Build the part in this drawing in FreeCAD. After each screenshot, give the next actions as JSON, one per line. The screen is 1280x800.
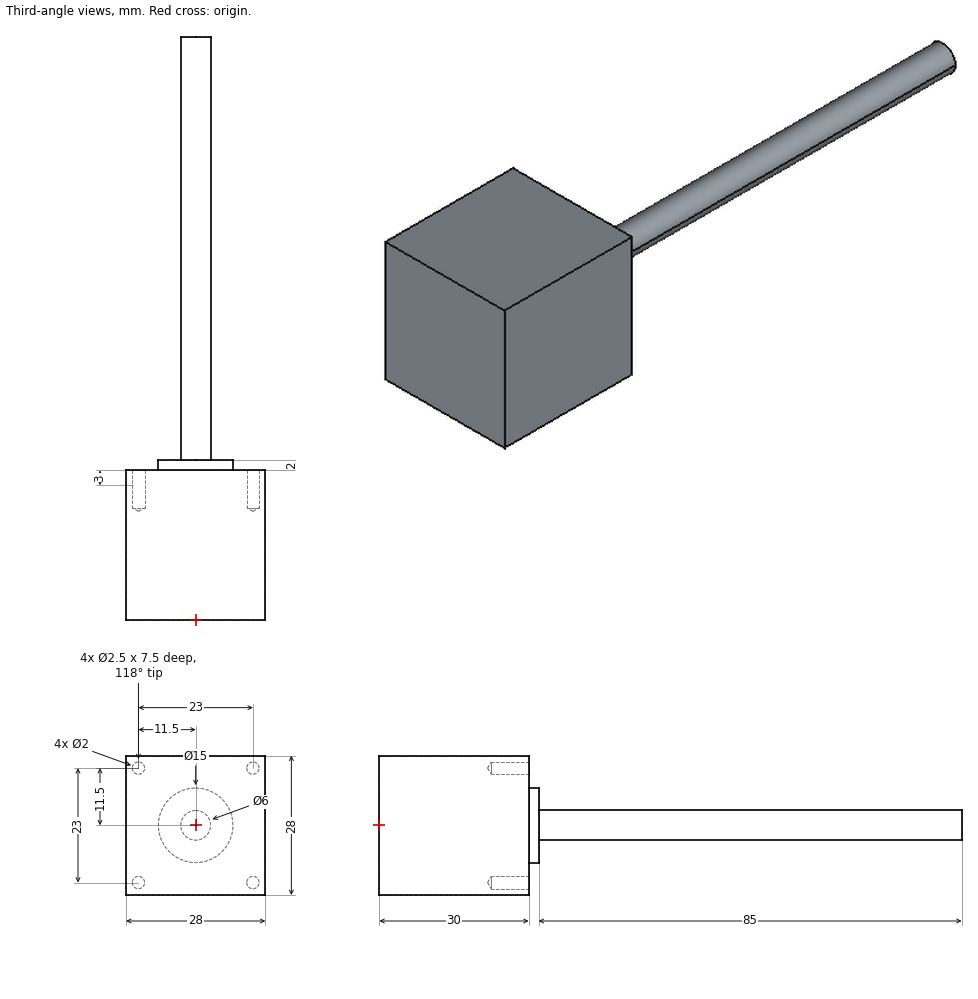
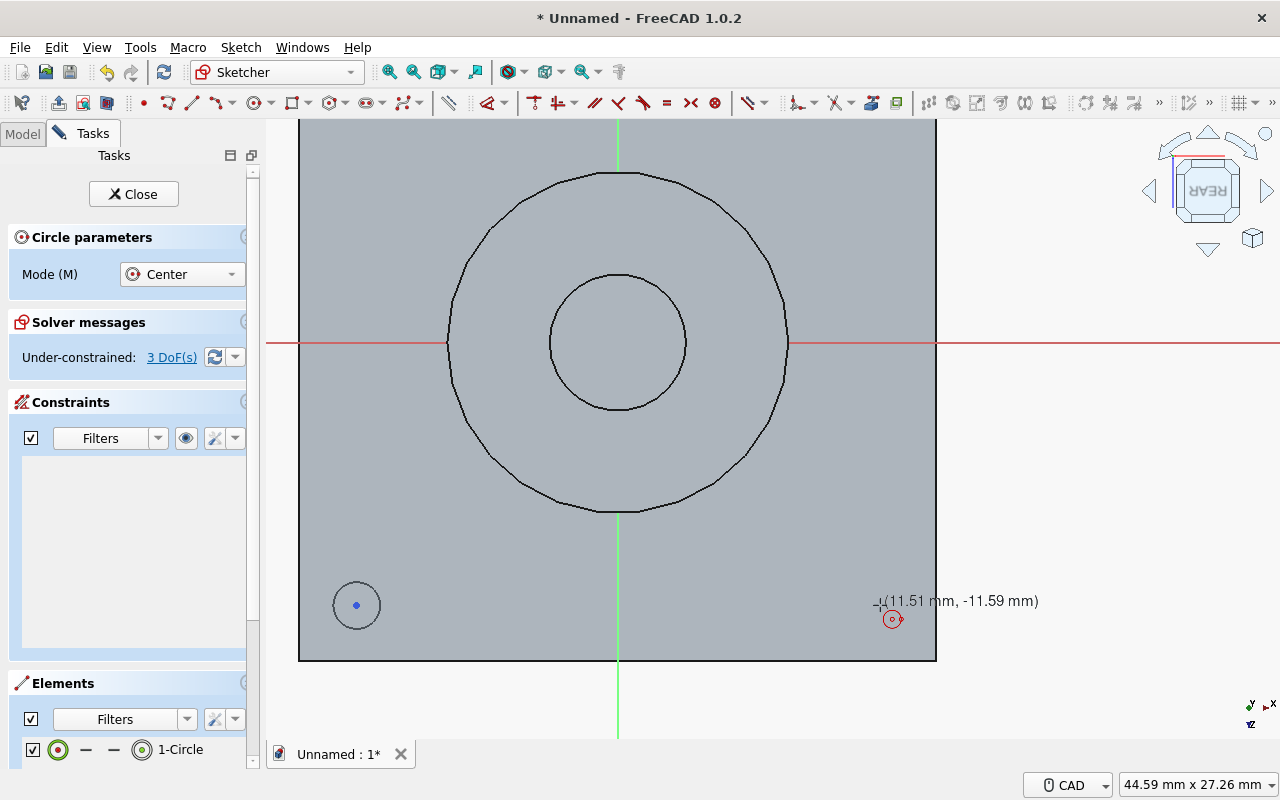
{"action": "left_click", "coordinate": [879, 604]}
{"action": "left_click", "coordinate": [895, 588]}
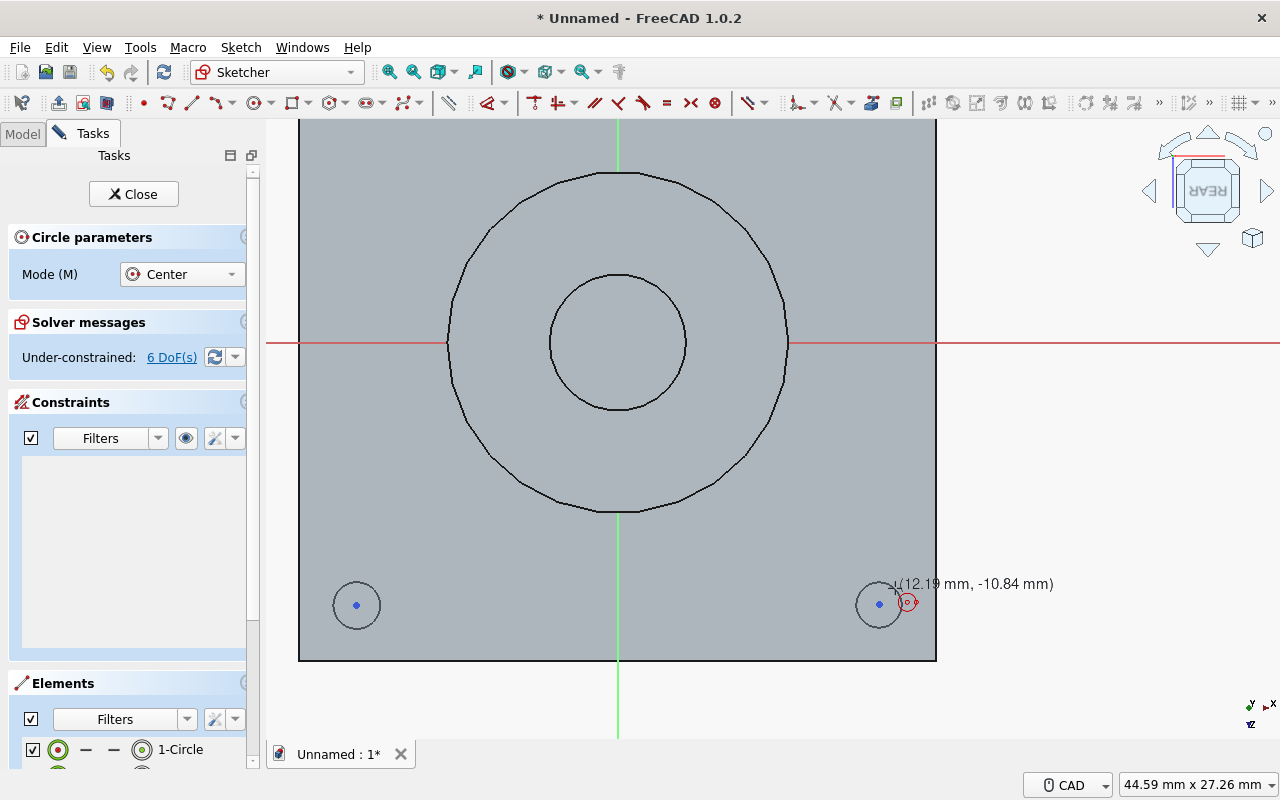
{"action": "scroll", "coordinate": [881, 605], "scroll_direction": "down", "scroll_amount": 2}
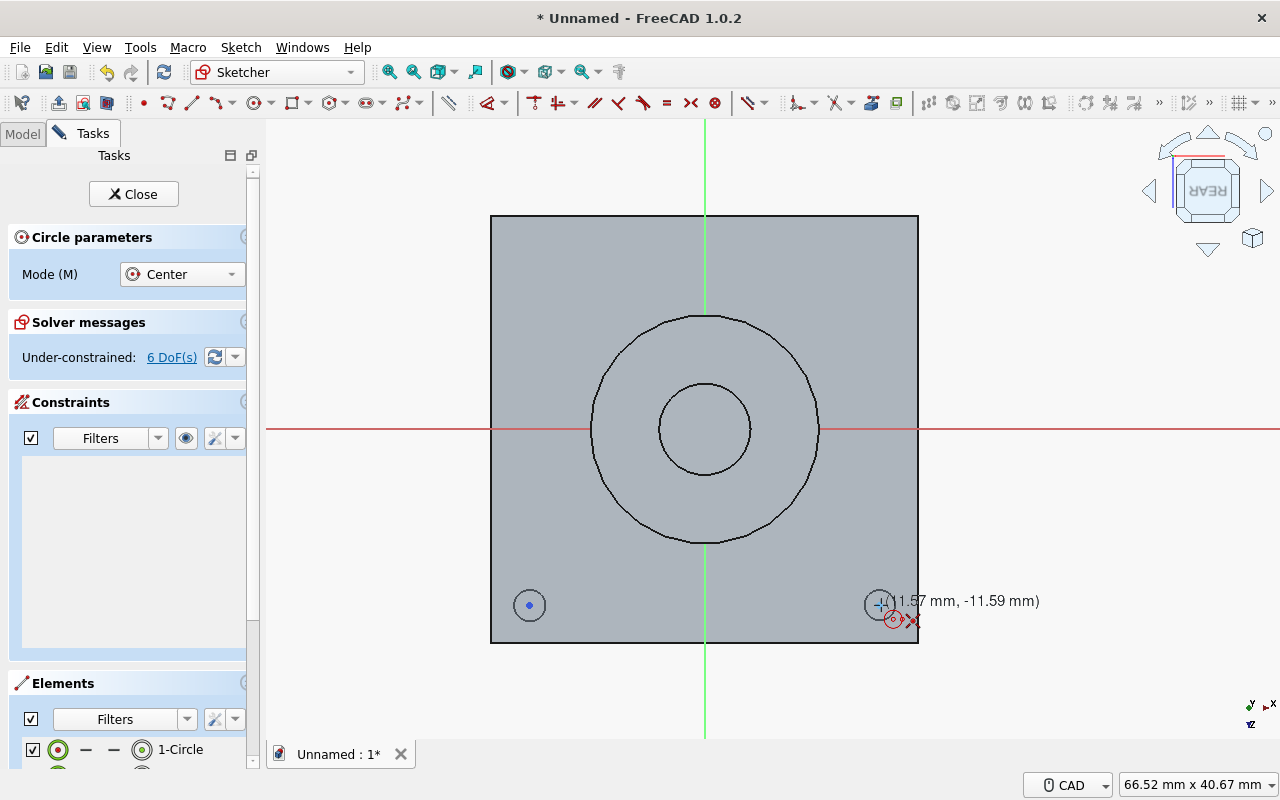
{"action": "scroll", "coordinate": [530, 254], "scroll_direction": "up", "scroll_amount": 2}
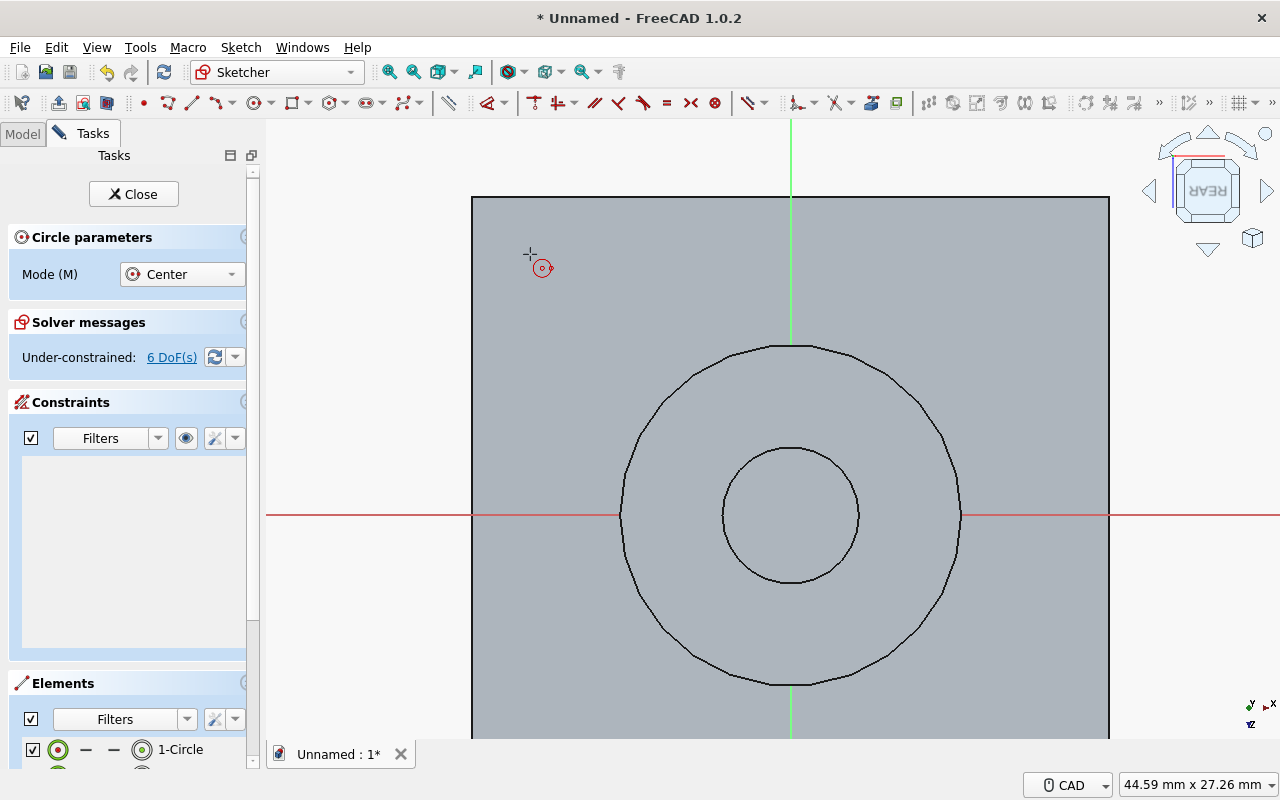
{"action": "left_click", "coordinate": [529, 254]}
{"action": "left_click", "coordinate": [545, 238]}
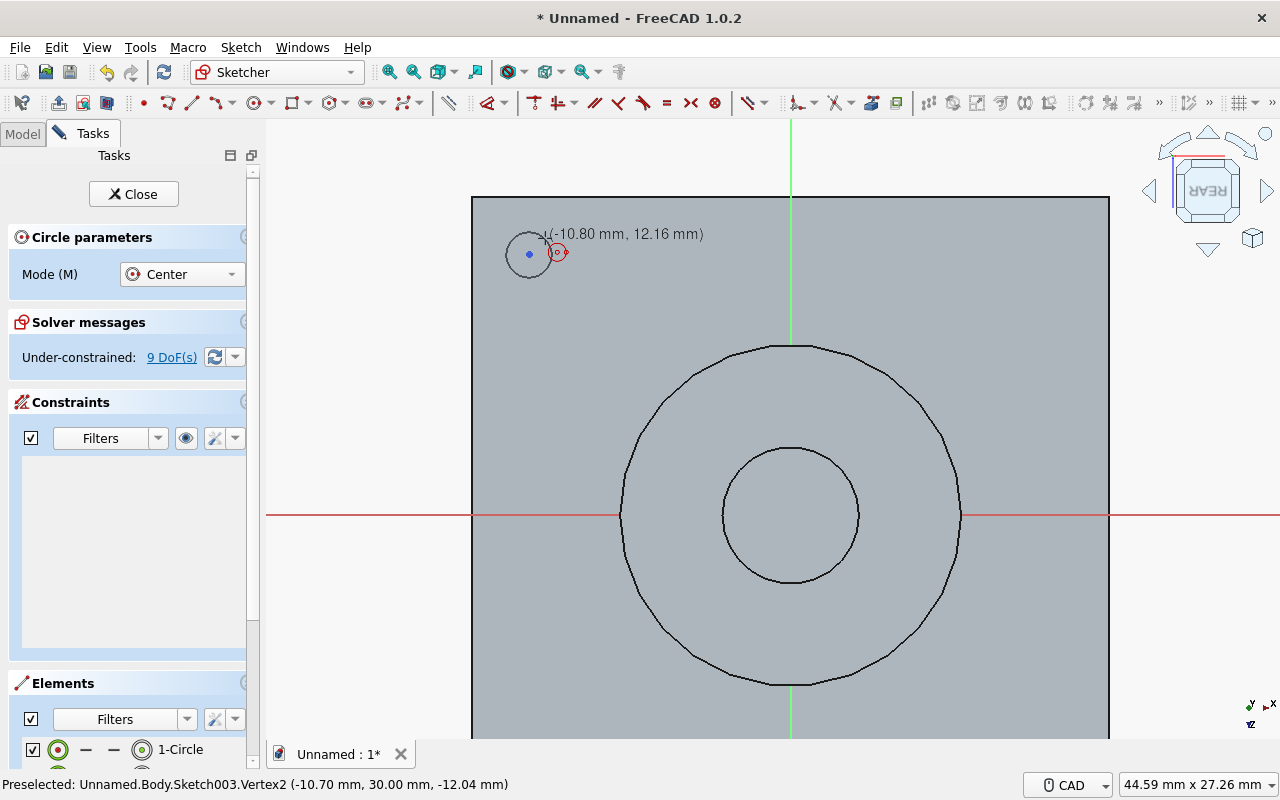
{"action": "left_click", "coordinate": [1052, 254]}
{"action": "left_click", "coordinate": [1068, 238]}
{"action": "key", "text": "Escape"}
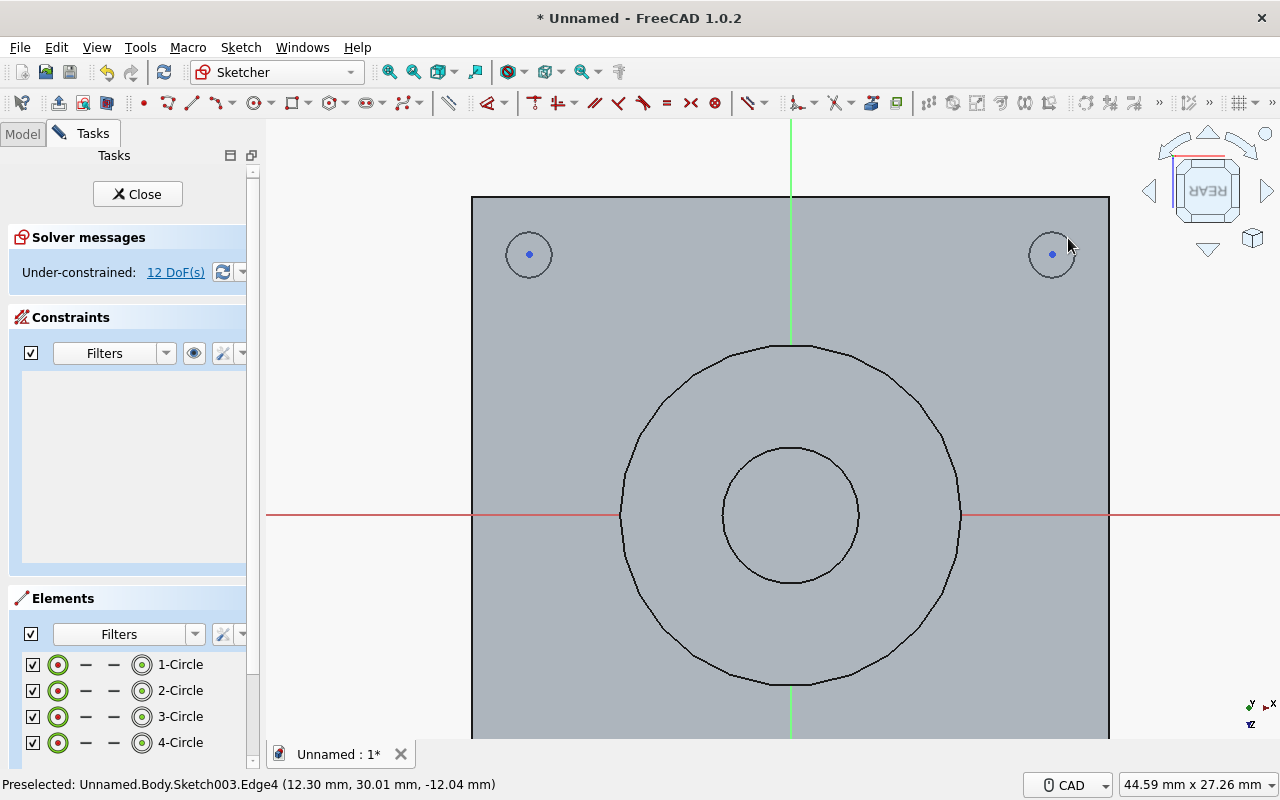
{"action": "scroll", "coordinate": [529, 253], "scroll_direction": "down", "scroll_amount": 2}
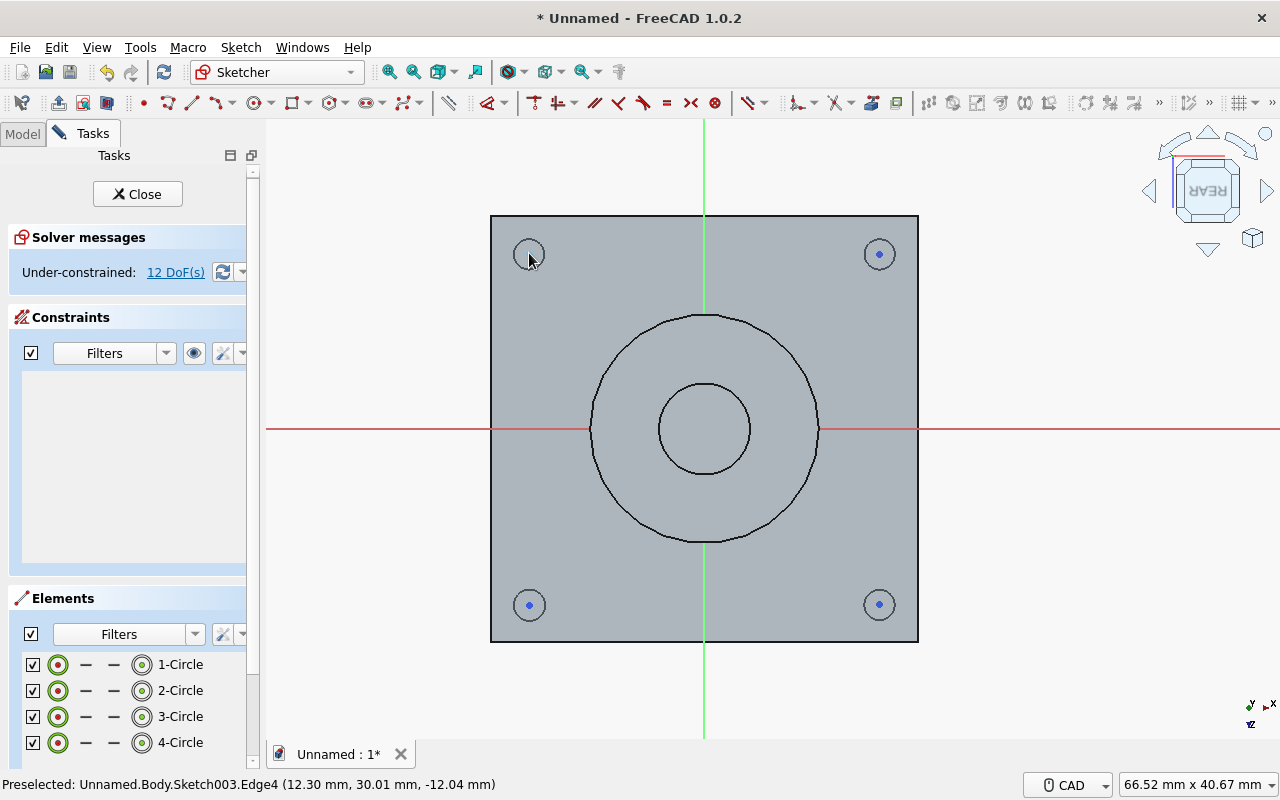
{"action": "left_click", "coordinate": [540, 594]}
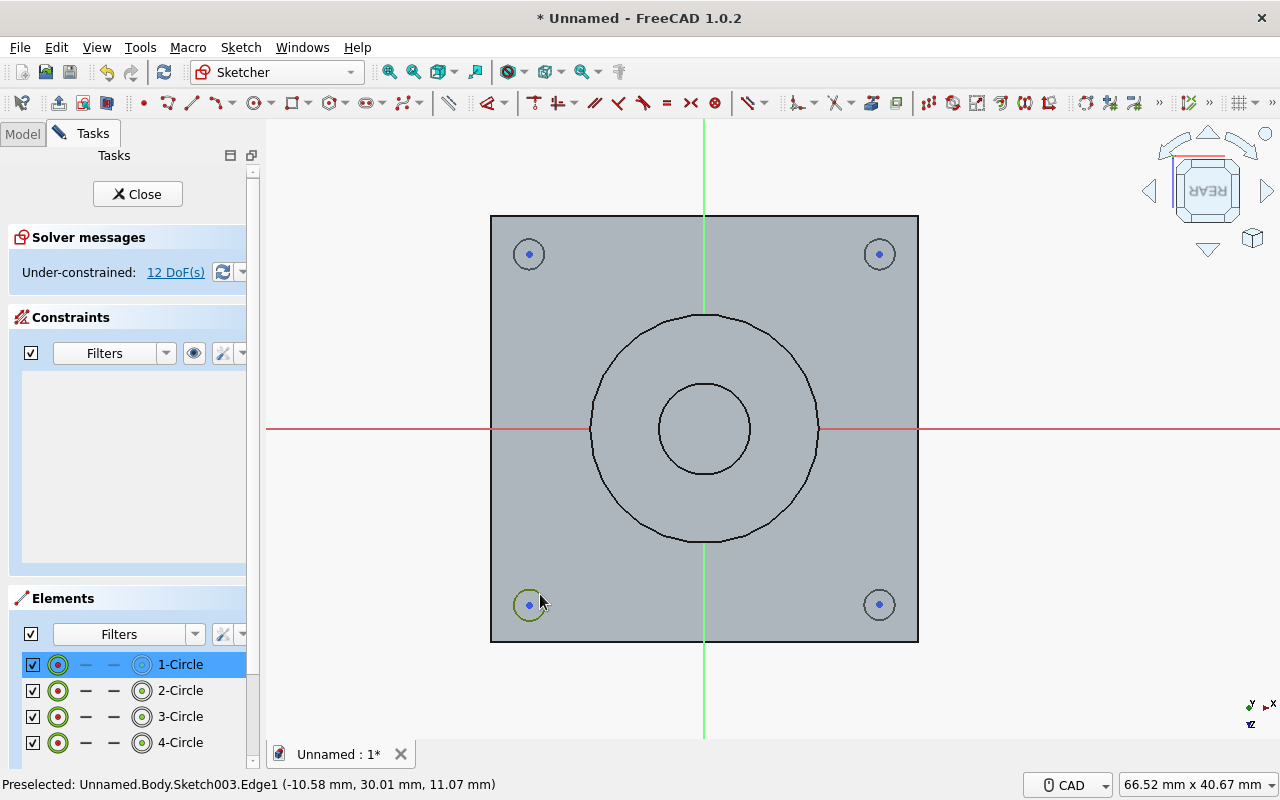
{"action": "left_click", "coordinate": [890, 594]}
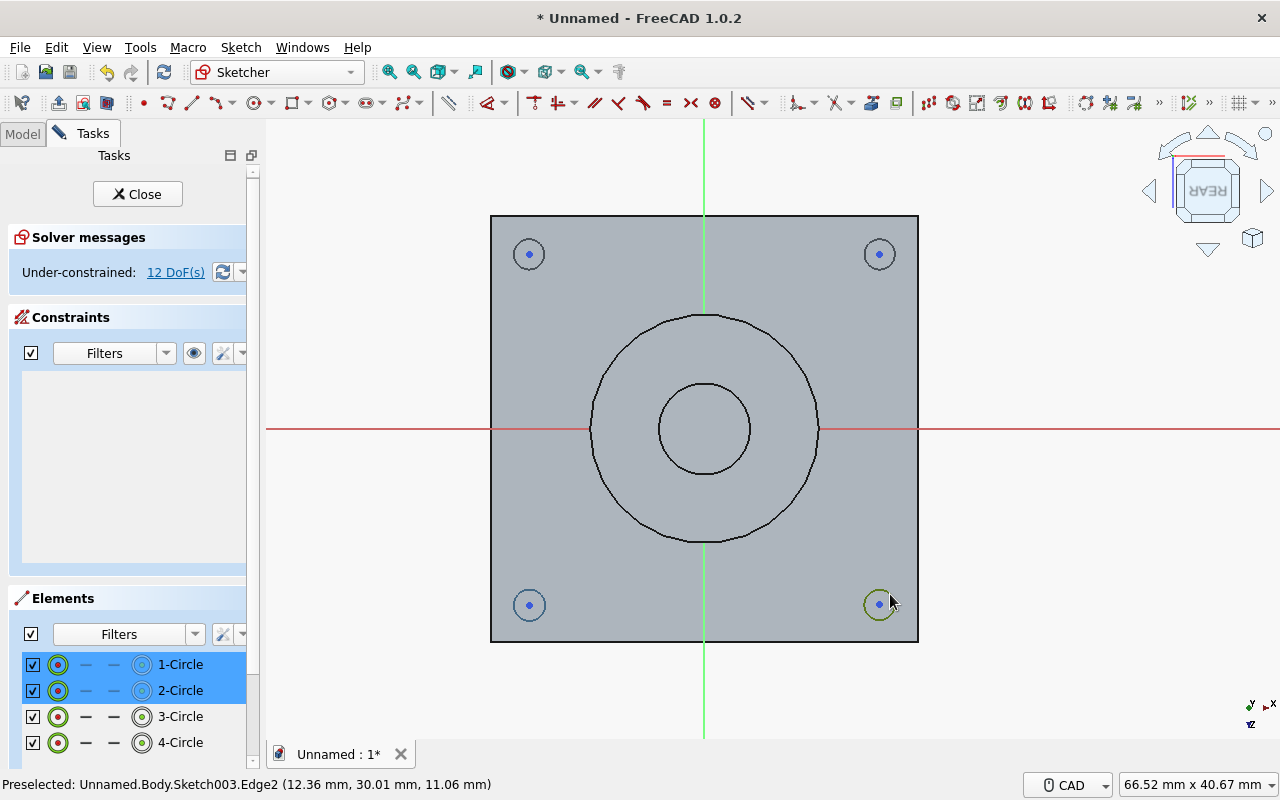
{"action": "left_click", "coordinate": [540, 244]}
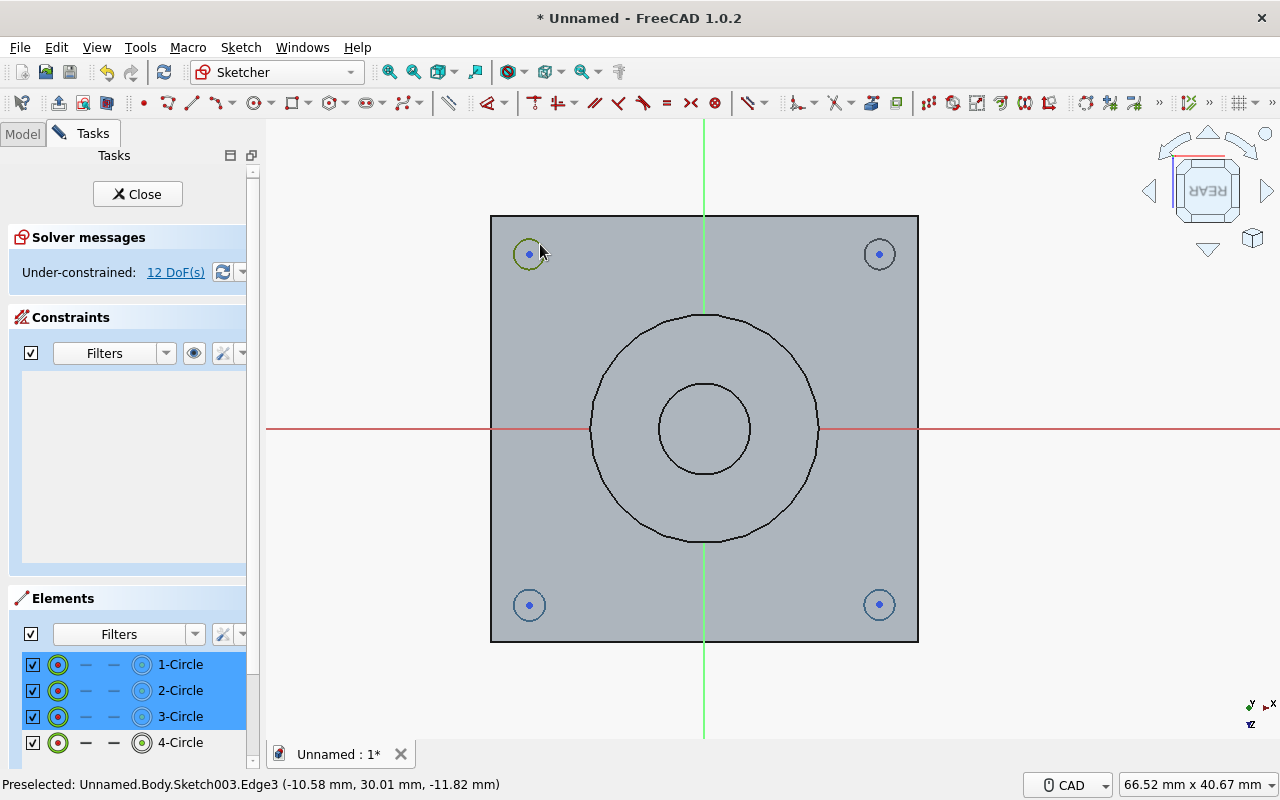
{"action": "left_click", "coordinate": [890, 244]}